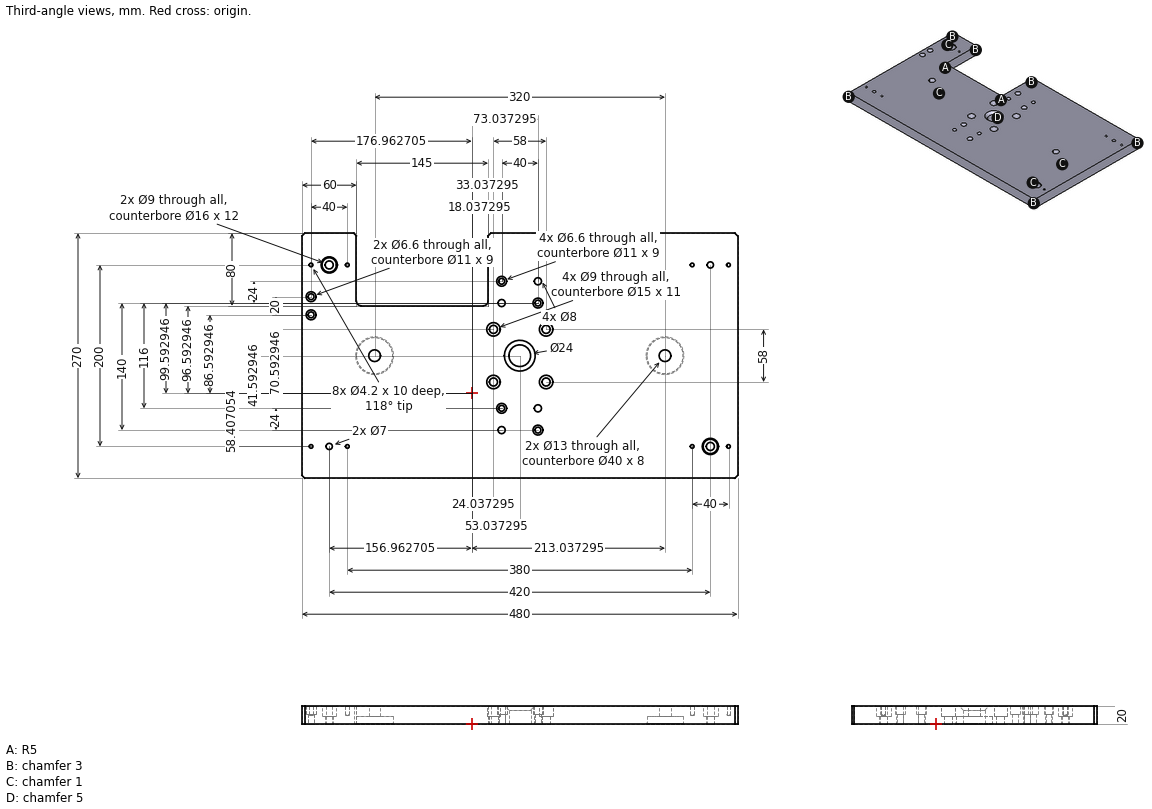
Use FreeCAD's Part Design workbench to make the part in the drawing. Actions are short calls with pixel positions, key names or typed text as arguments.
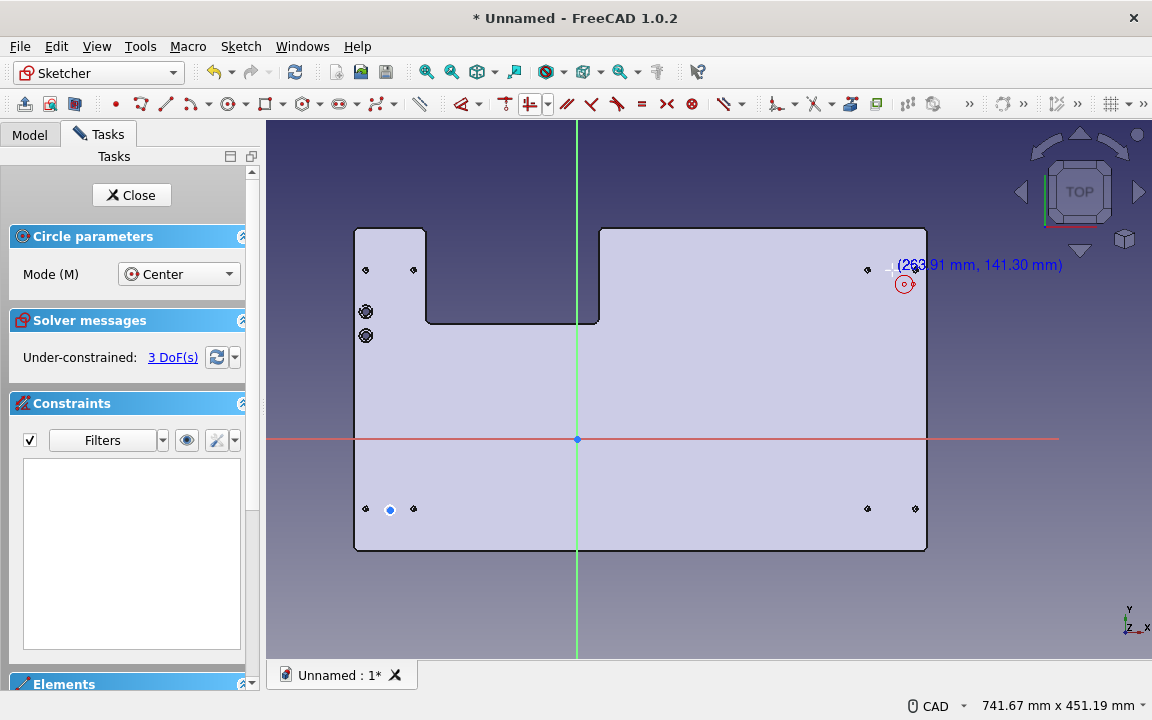
click(892, 270)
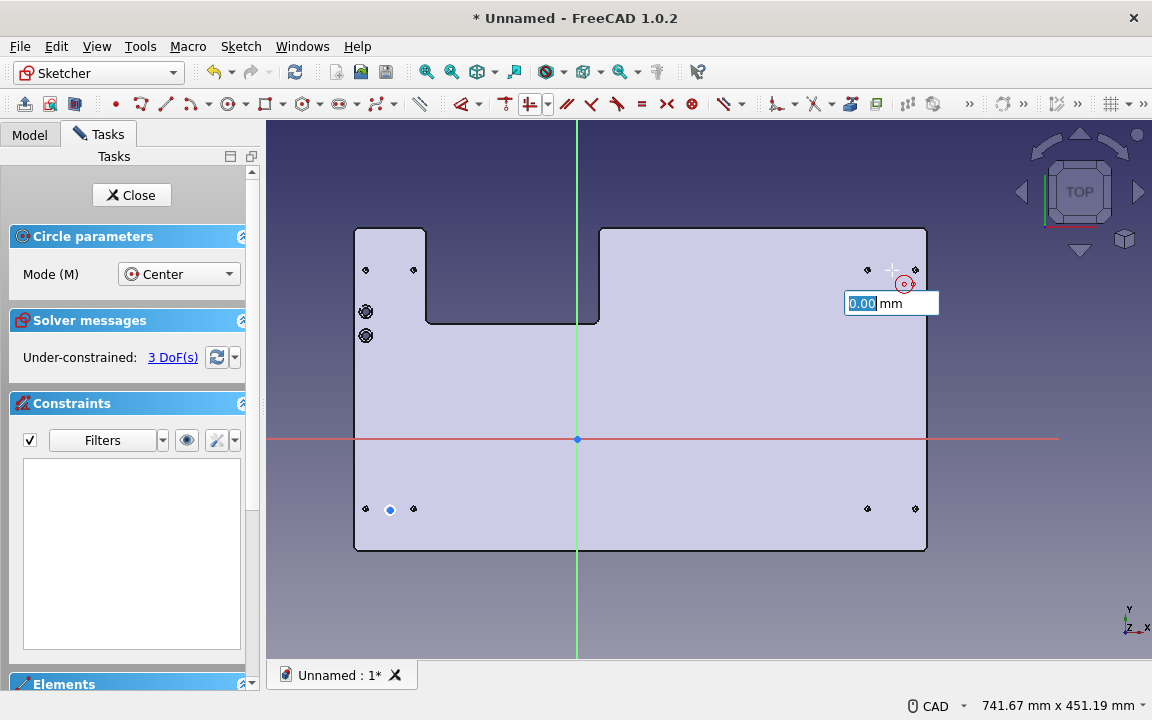
scroll(895, 267, up, 7)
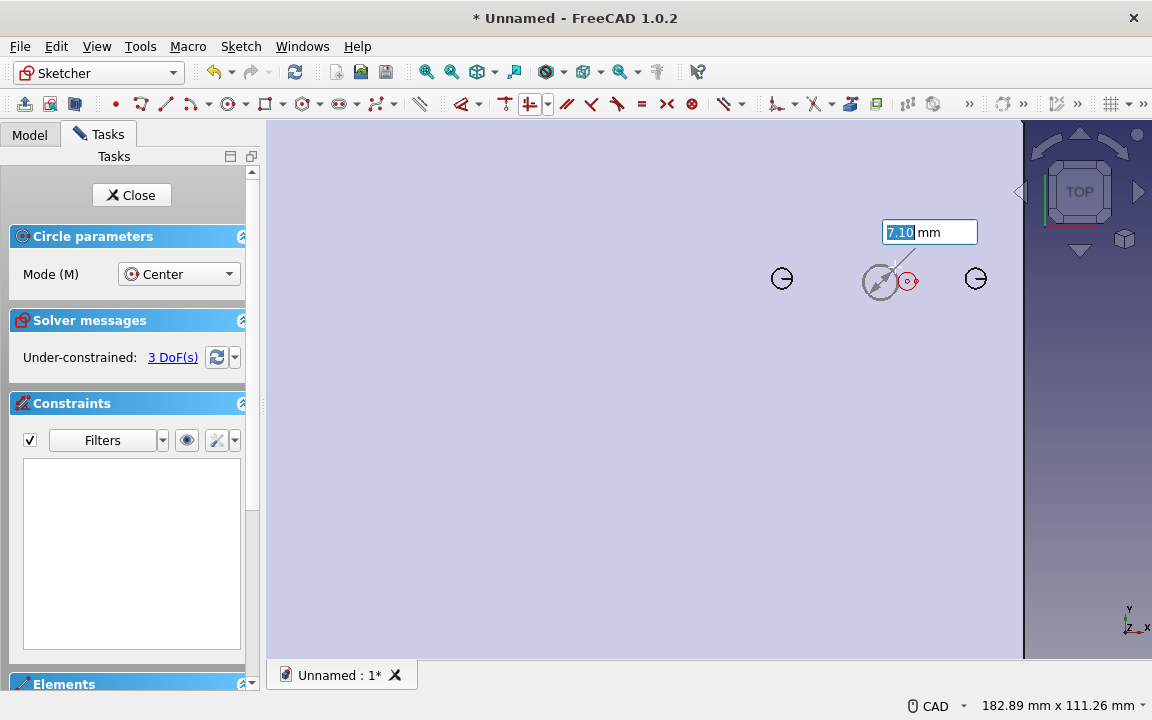
click(891, 267)
key(Escape)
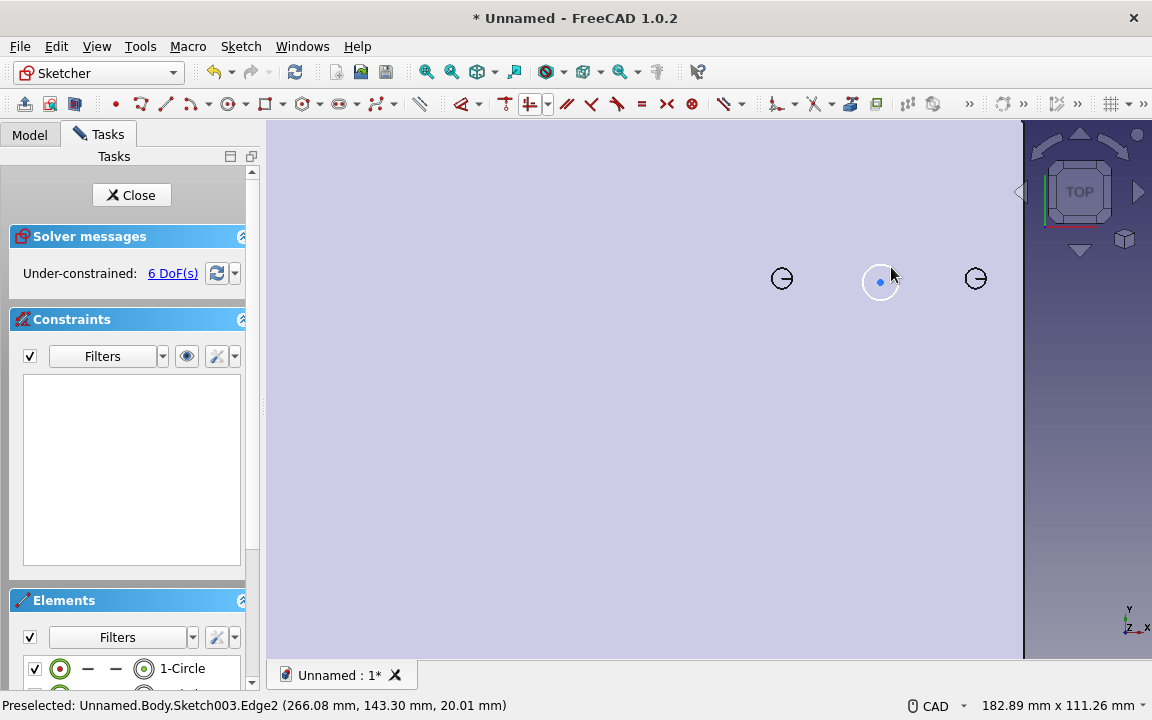
scroll(895, 267, down, 7)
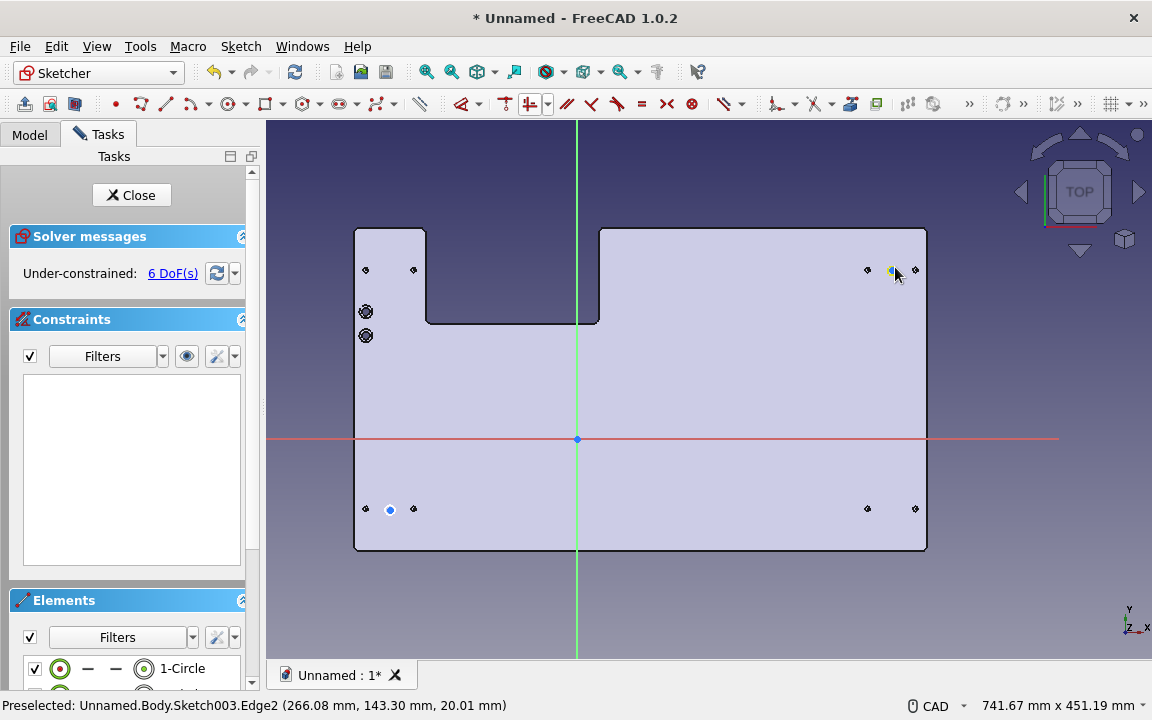
scroll(393, 507, up, 6)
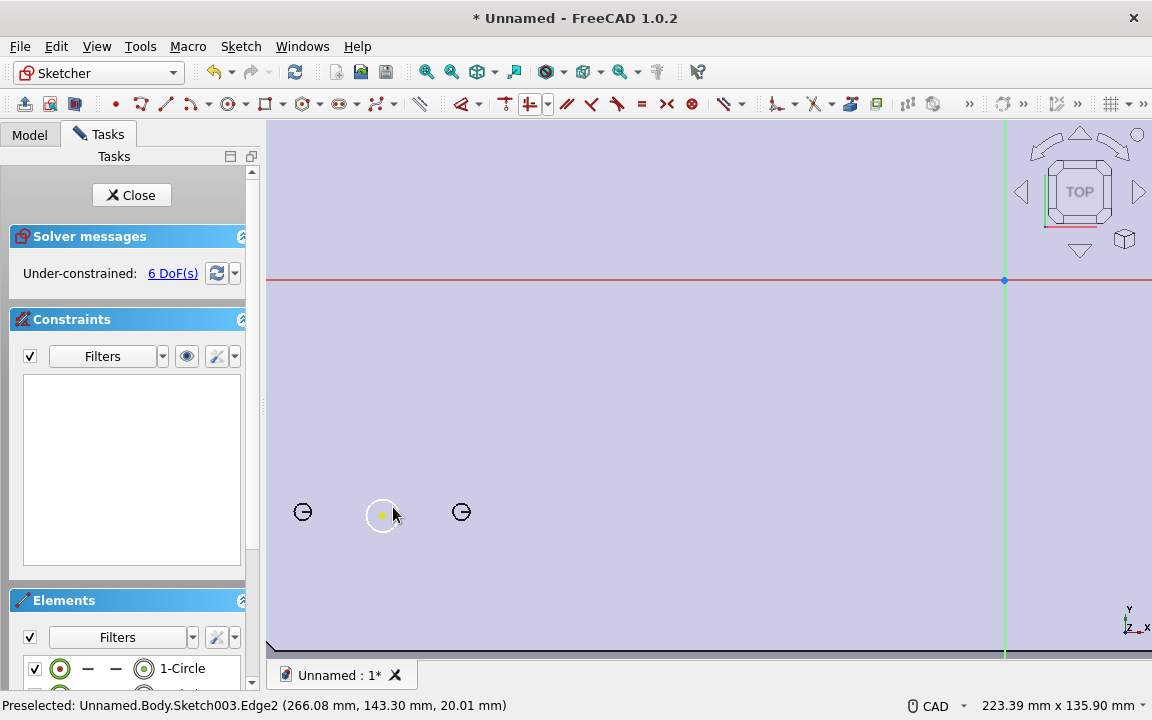
click(394, 504)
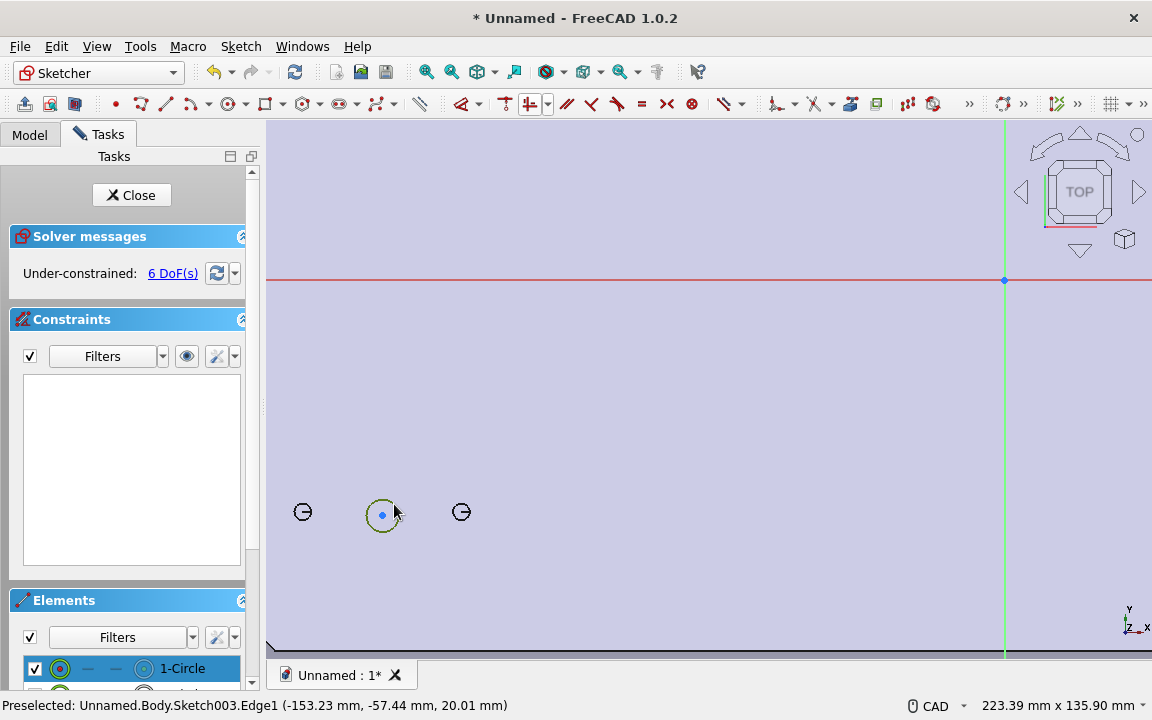
scroll(393, 508, down, 6)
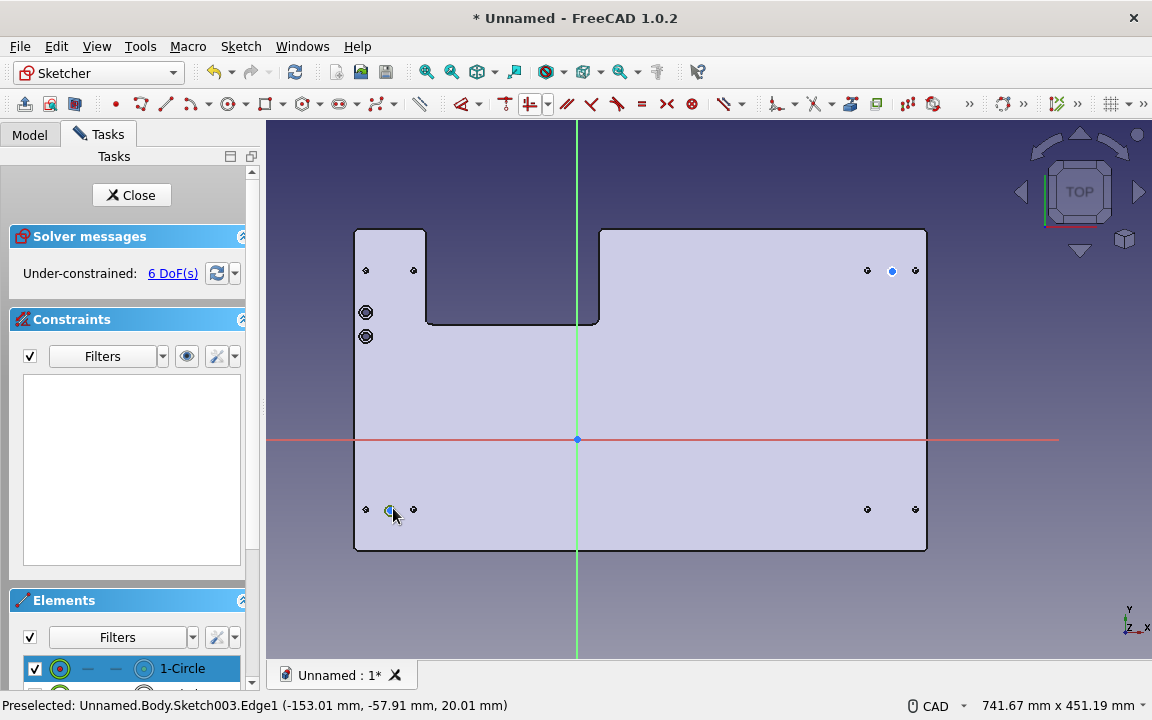
scroll(895, 269, up, 6)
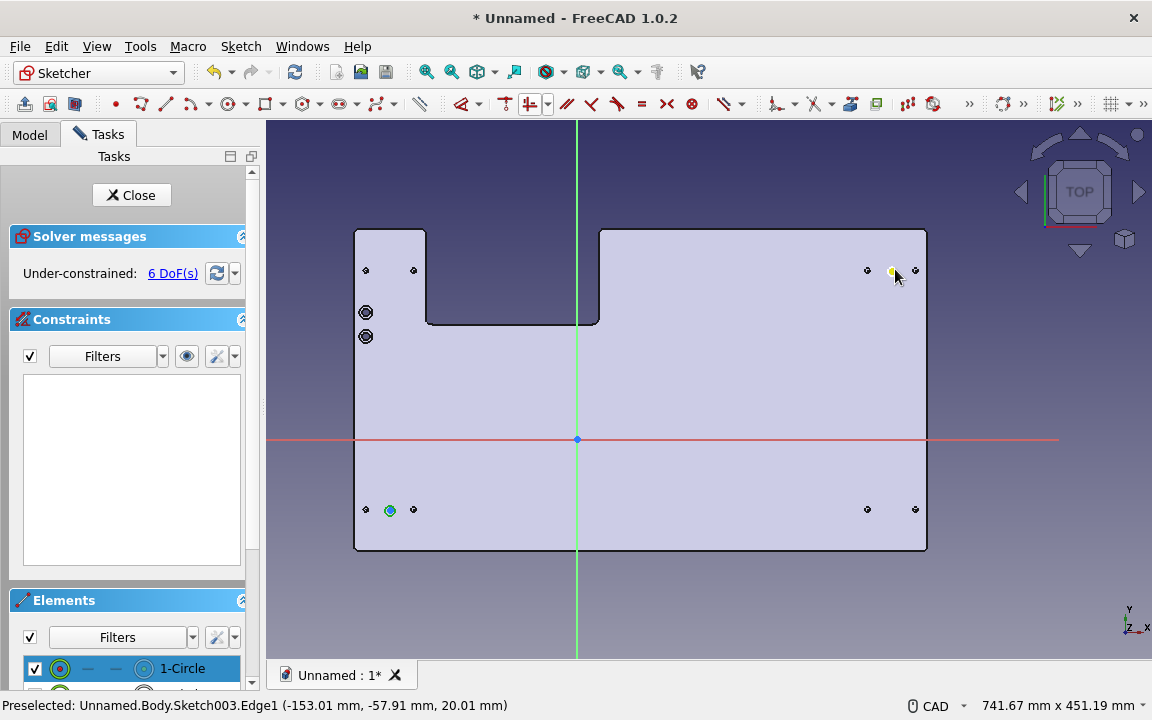
click(894, 267)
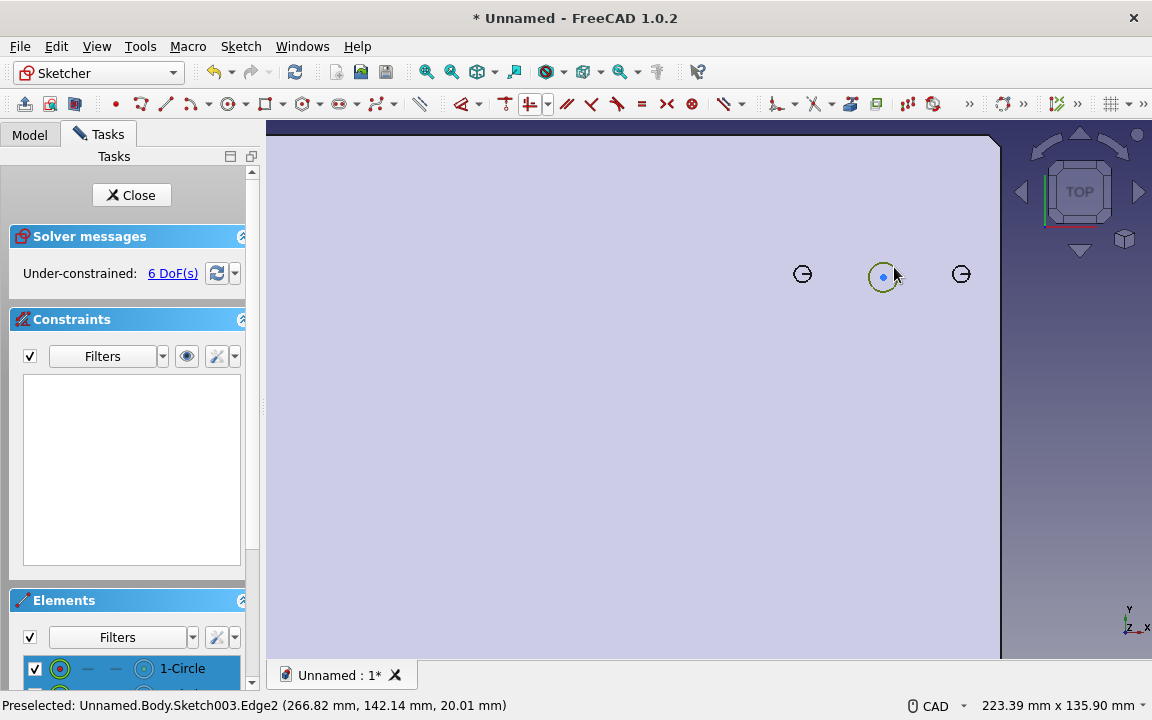
click(642, 104)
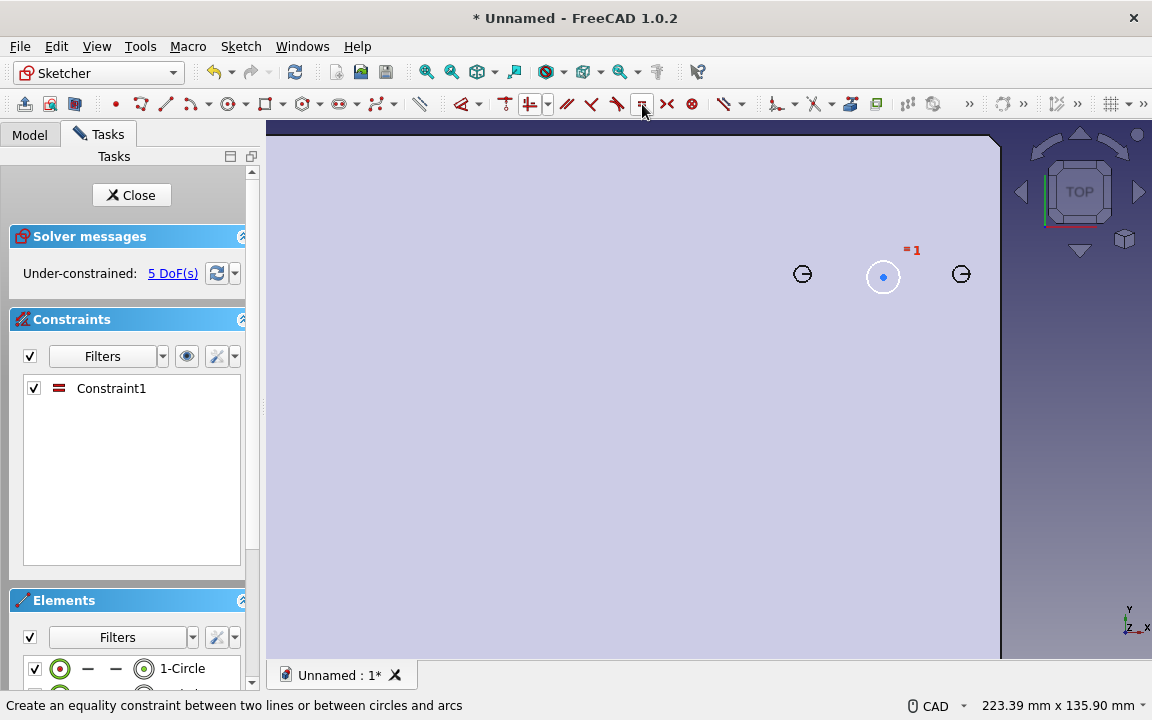
click(460, 104)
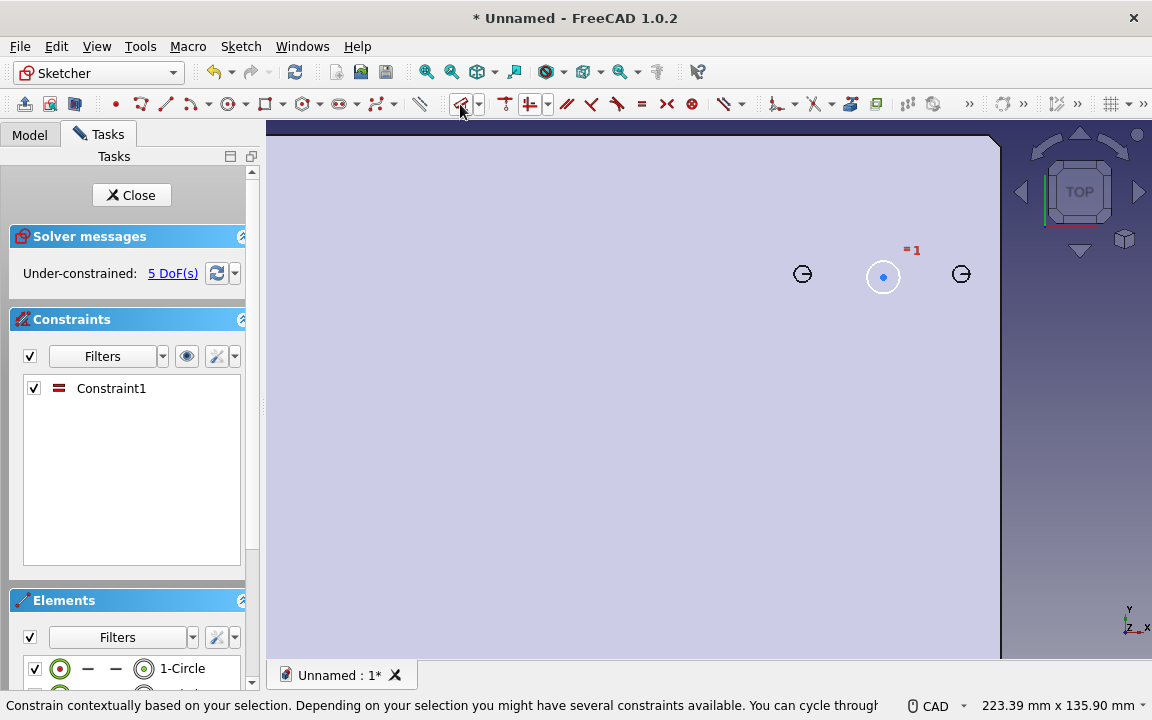
scroll(895, 268, down, 6)